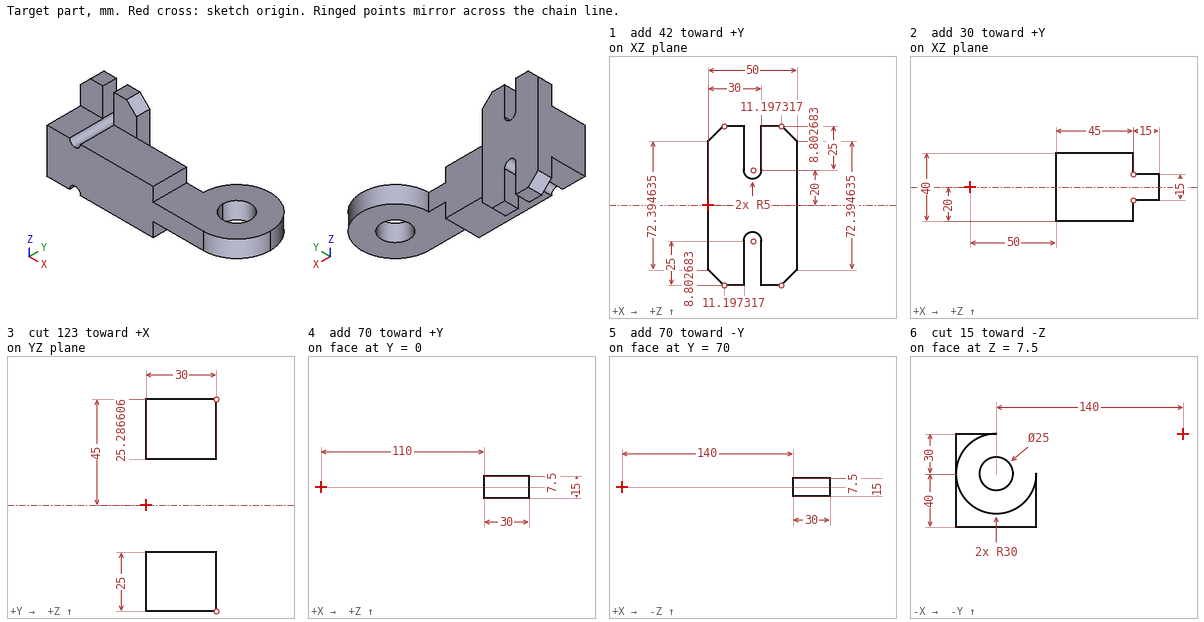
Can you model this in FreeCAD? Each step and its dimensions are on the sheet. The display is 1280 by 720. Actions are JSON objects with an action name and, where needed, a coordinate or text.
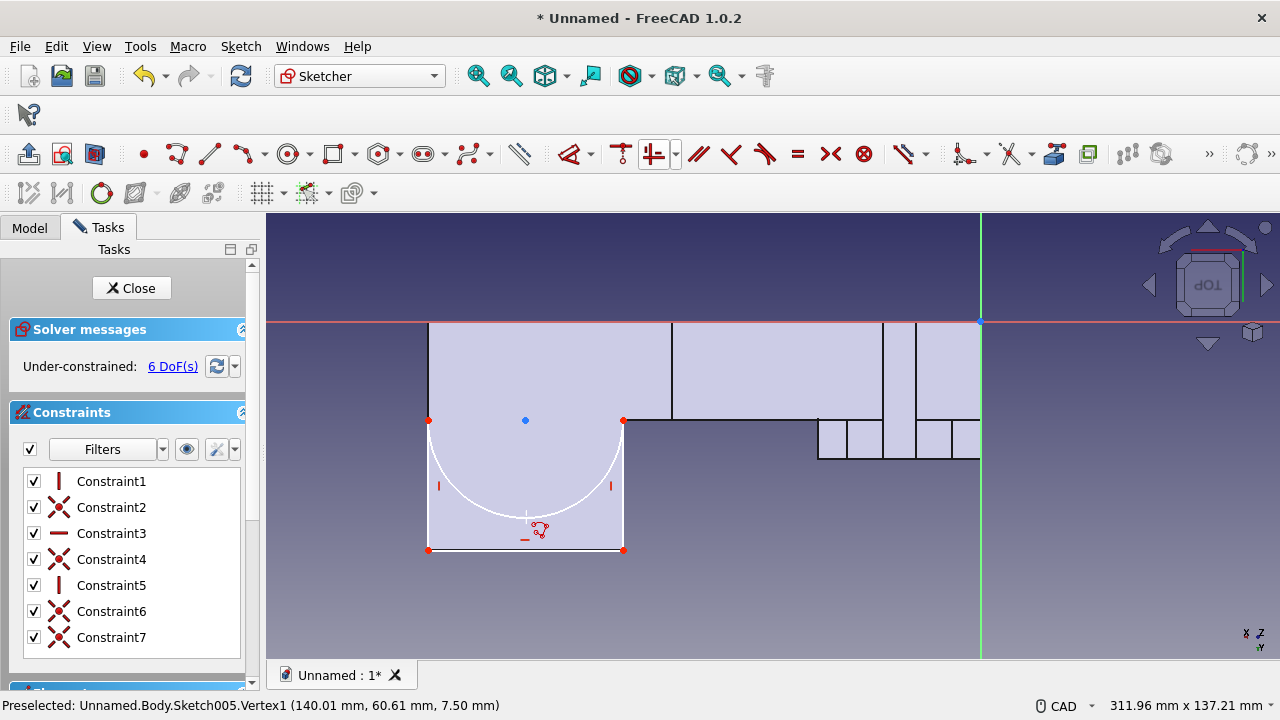
{"action": "left_click", "coordinate": [526, 322]}
{"action": "left_click", "coordinate": [428, 331]}
{"action": "left_click", "coordinate": [428, 421]}
{"action": "right_click", "coordinate": [428, 331]}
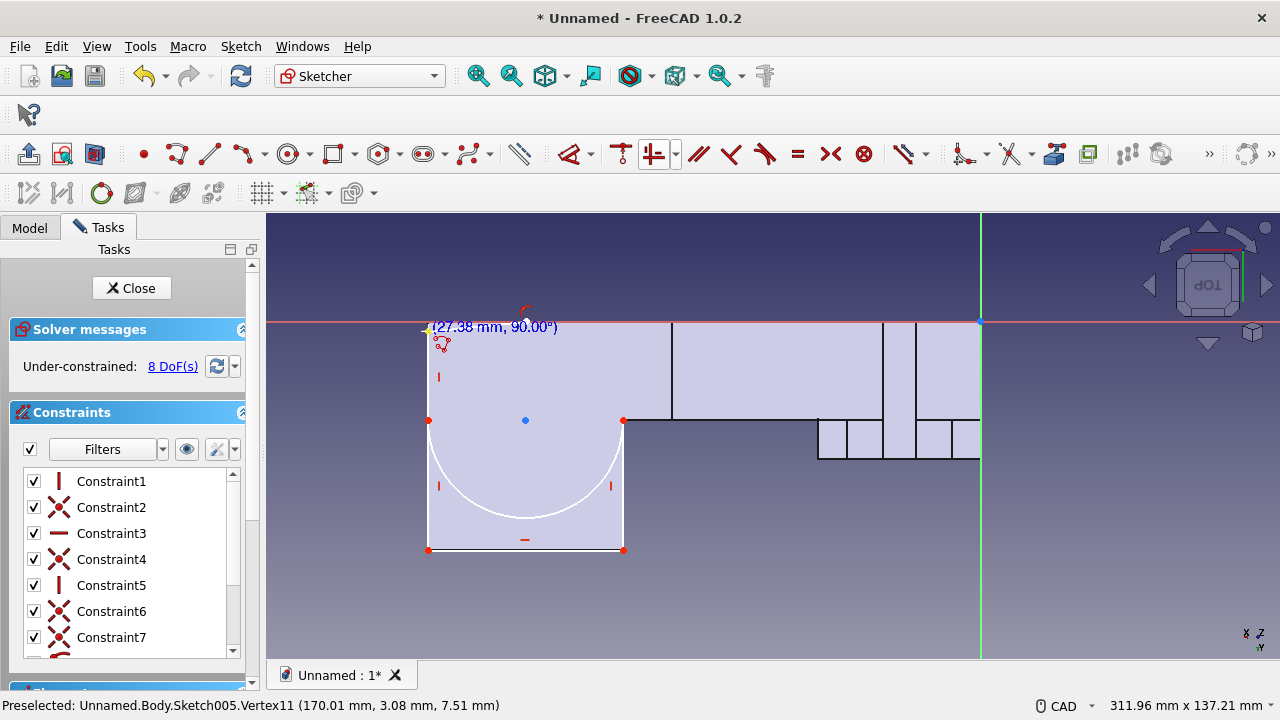
{"action": "left_click", "coordinate": [242, 154]}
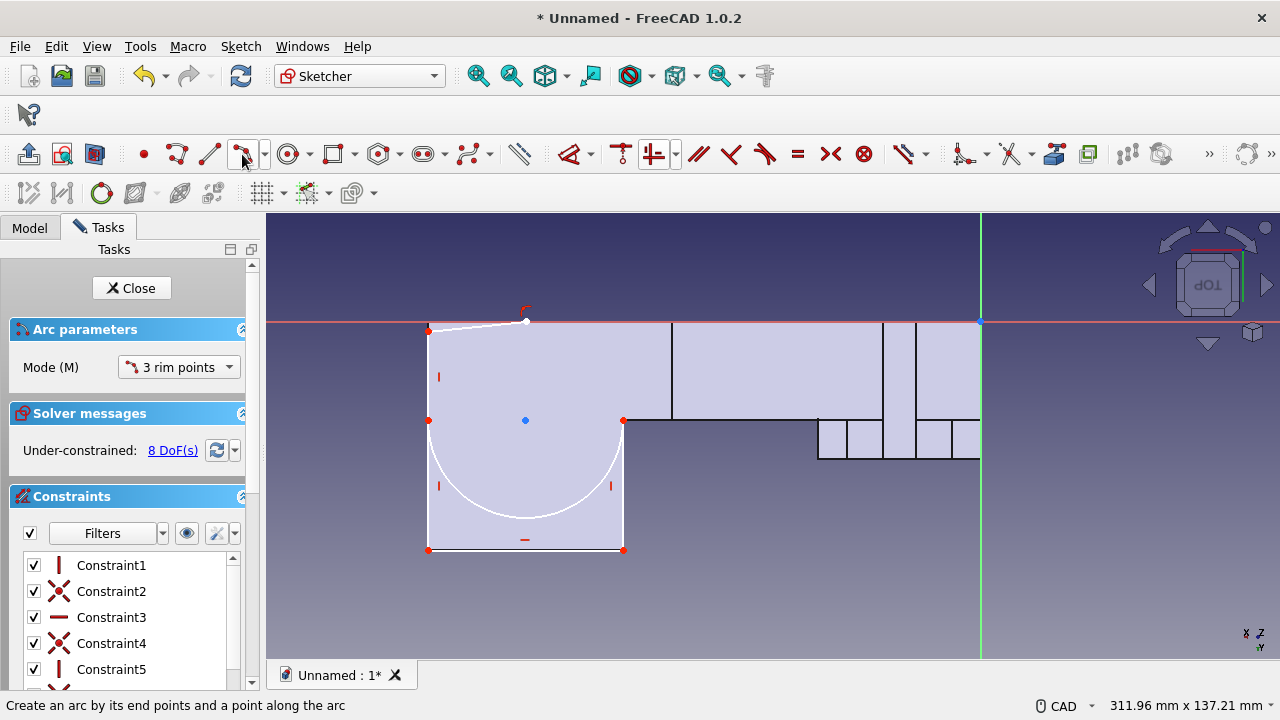
{"action": "left_click", "coordinate": [428, 421]}
{"action": "left_click", "coordinate": [526, 322]}
{"action": "left_click", "coordinate": [457, 351]}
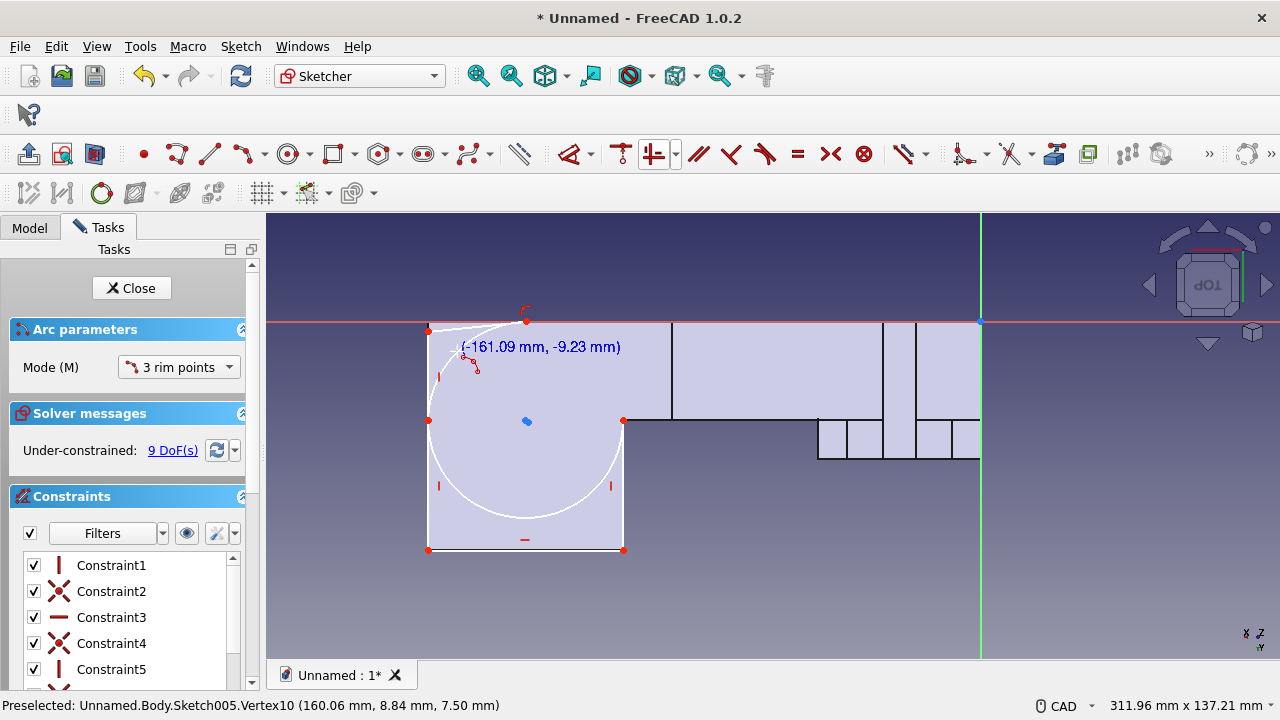
{"action": "left_click", "coordinate": [288, 154]}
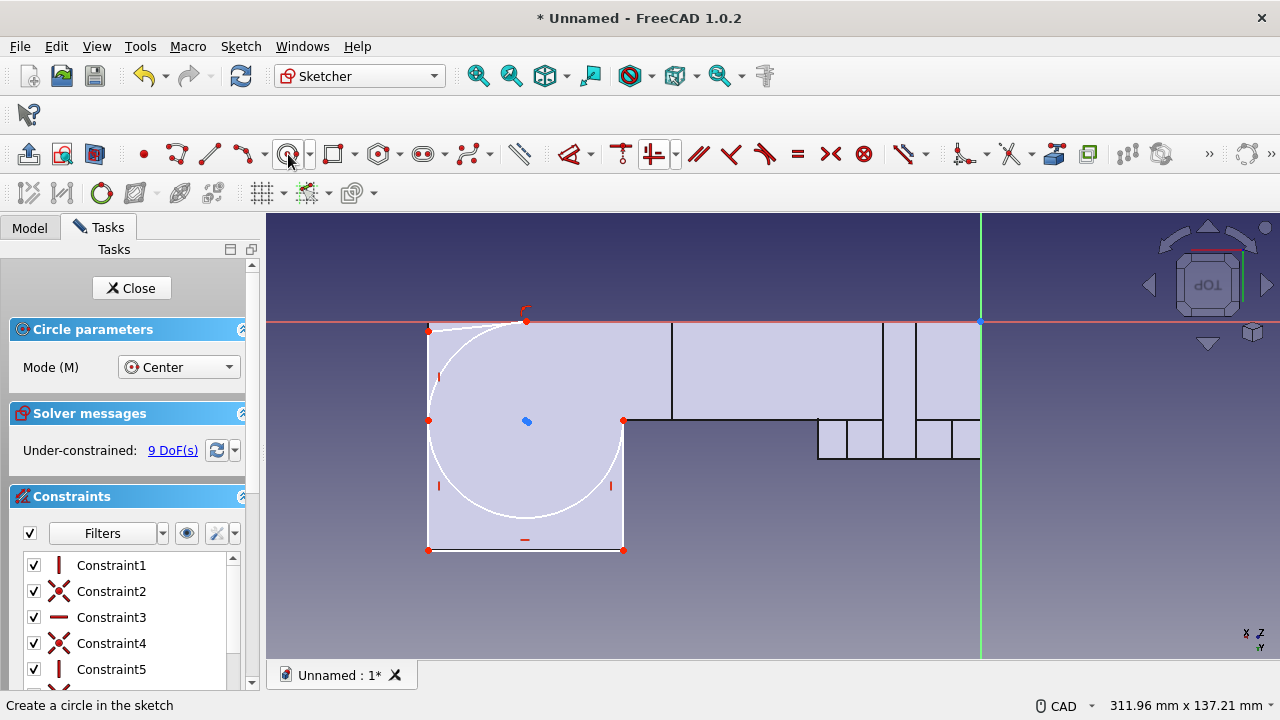
{"action": "left_click", "coordinate": [526, 420]}
{"action": "left_click", "coordinate": [554, 391]}
{"action": "key", "text": "Escape"}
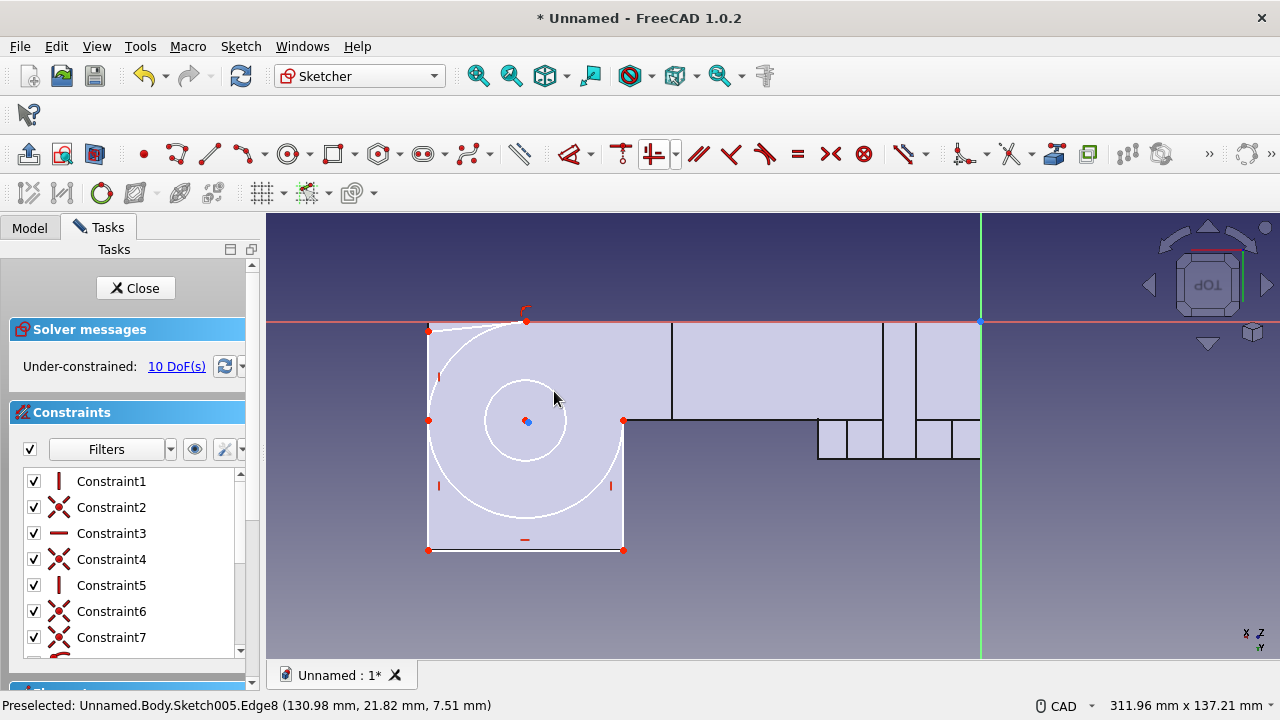
{"action": "left_click", "coordinate": [428, 512]}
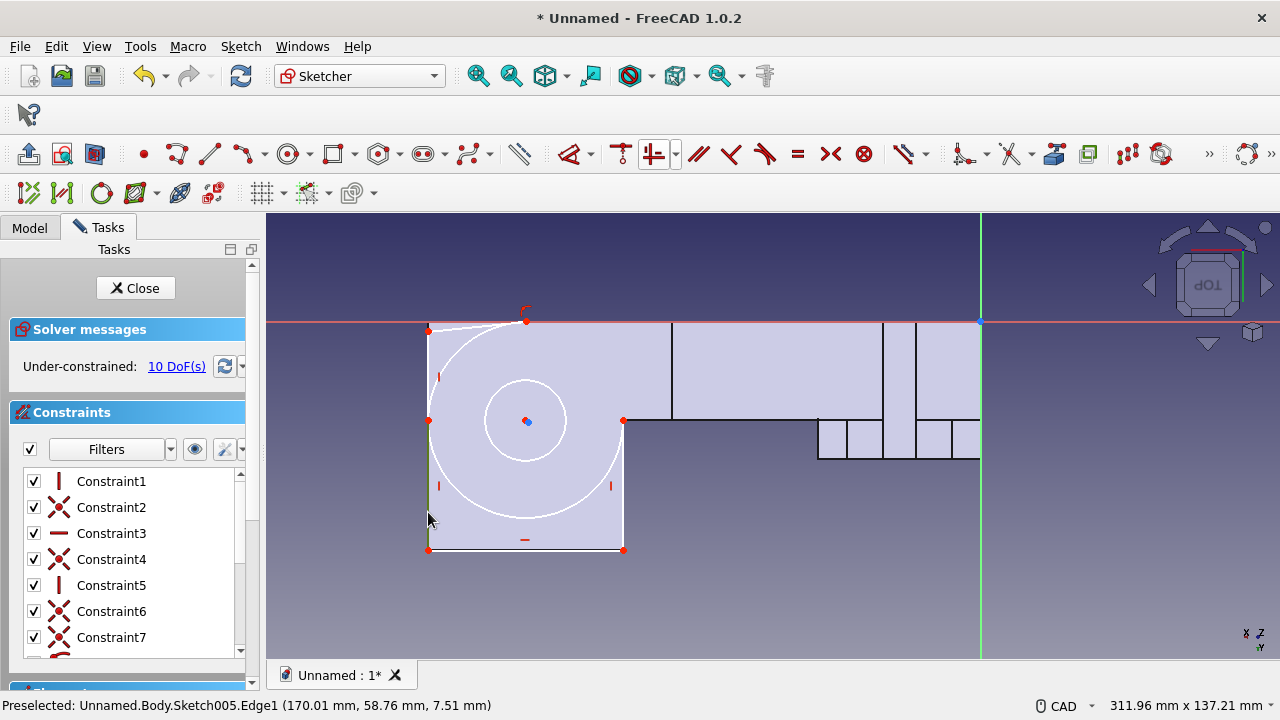
{"action": "left_click", "coordinate": [468, 499]}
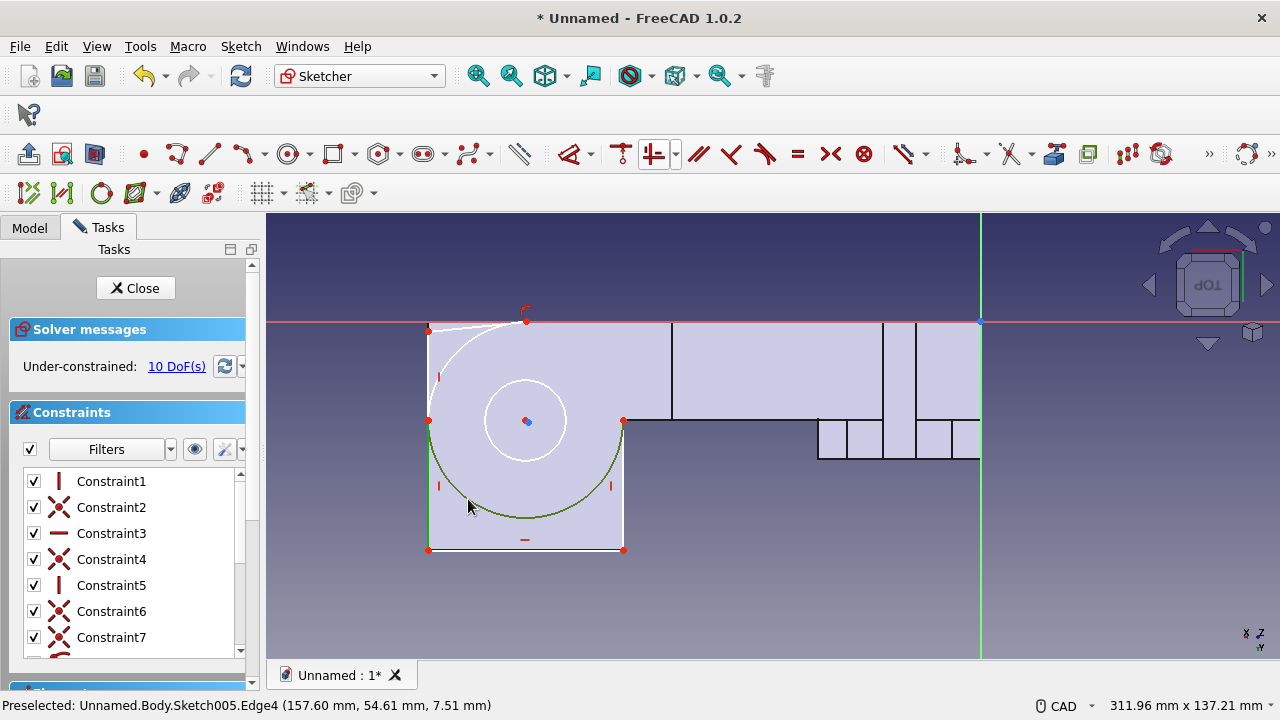
{"action": "left_click", "coordinate": [765, 154]}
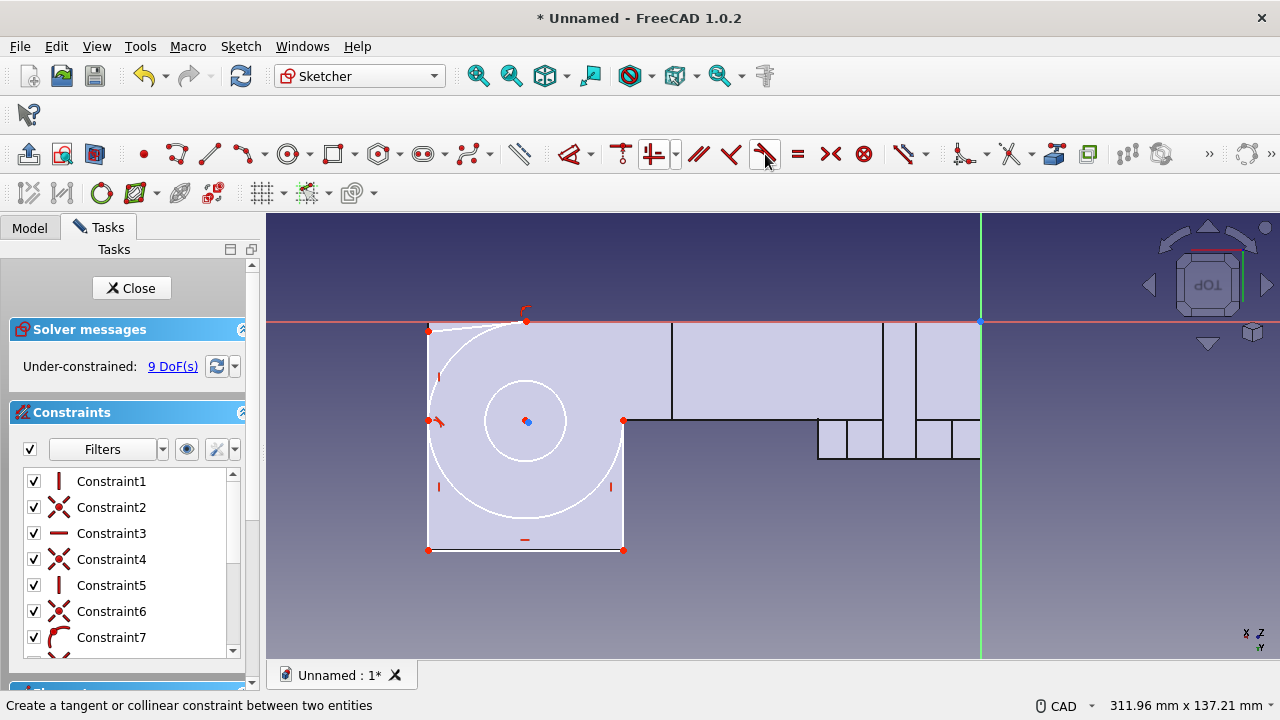
{"action": "left_click", "coordinate": [623, 512]}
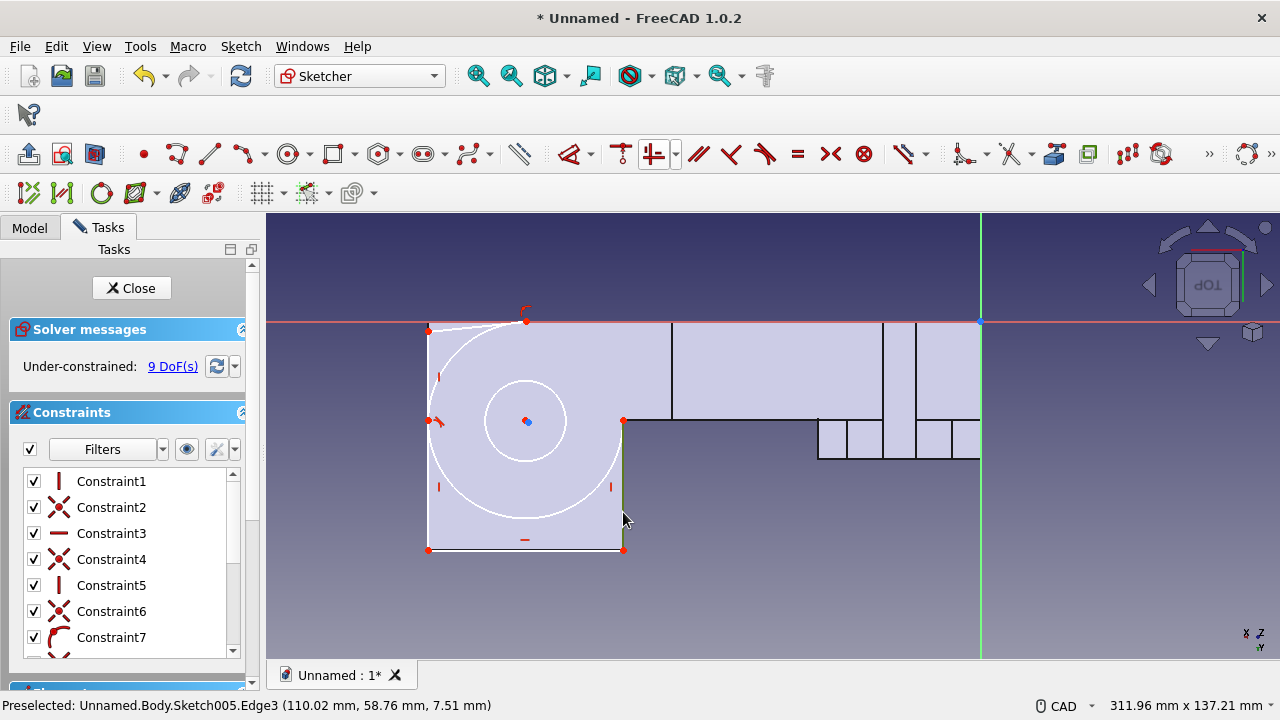
{"action": "left_click", "coordinate": [468, 500]}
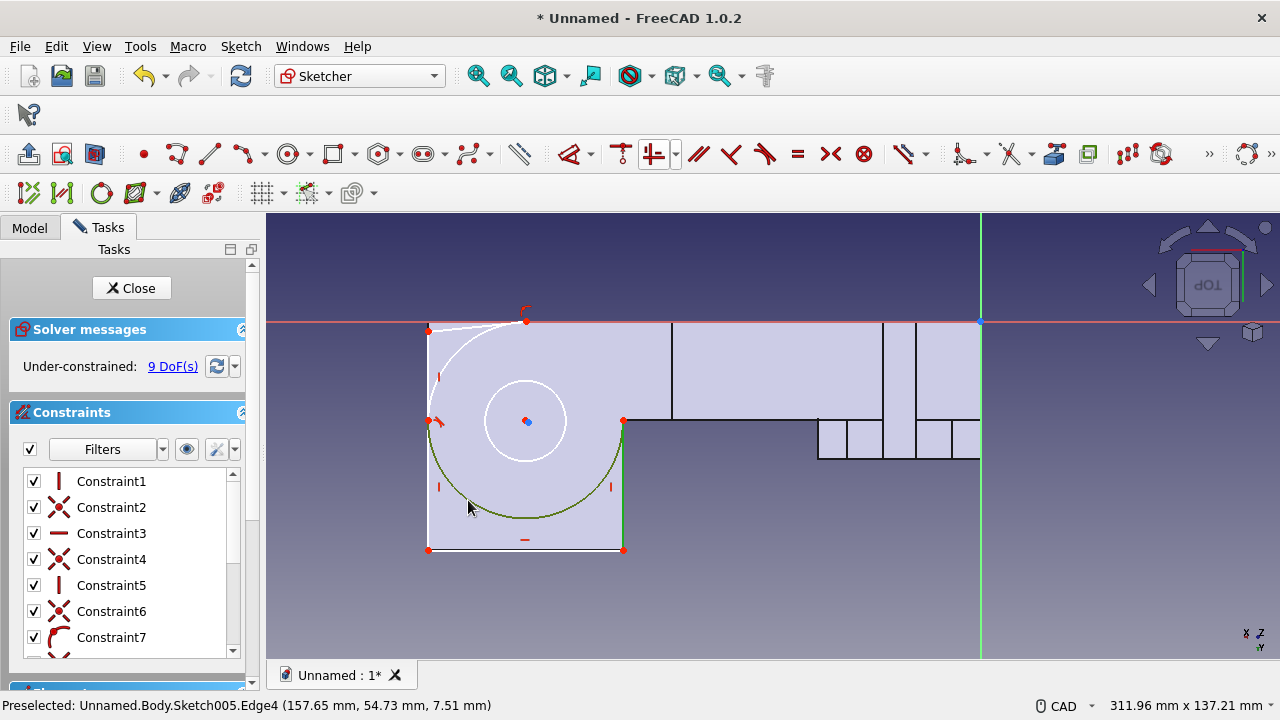
{"action": "left_click", "coordinate": [765, 154]}